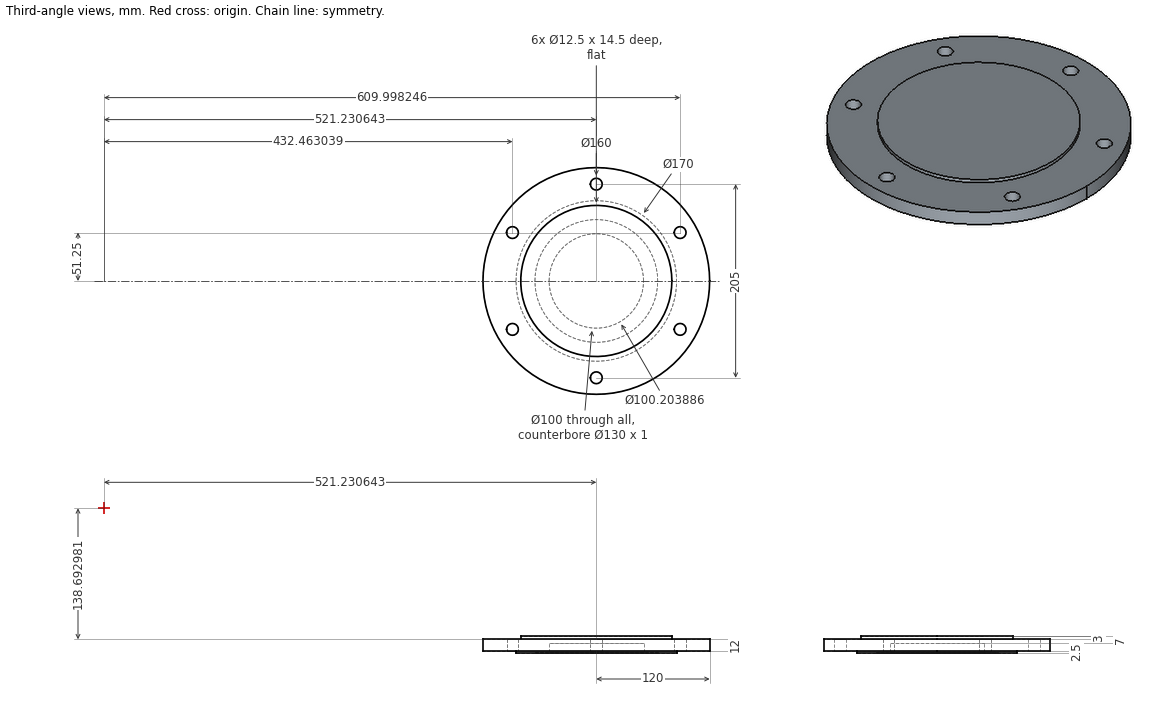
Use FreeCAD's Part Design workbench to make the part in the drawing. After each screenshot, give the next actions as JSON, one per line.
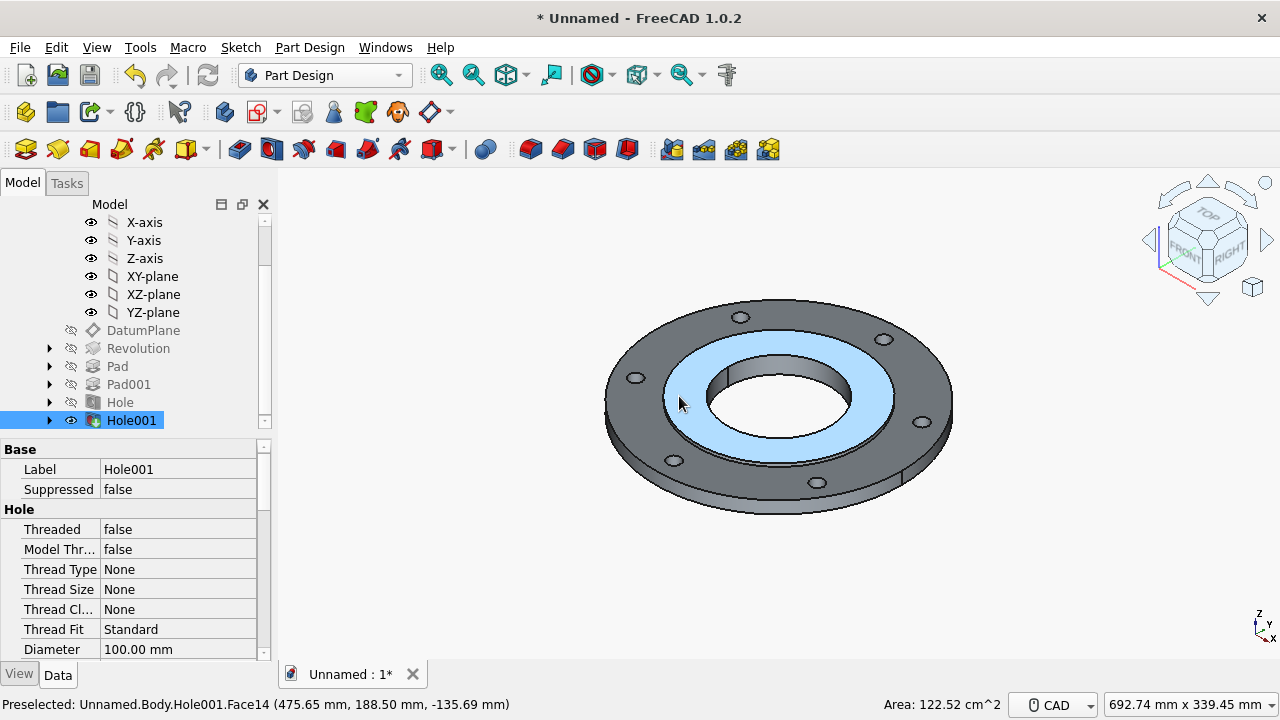
{"action": "left_click", "coordinate": [258, 112]}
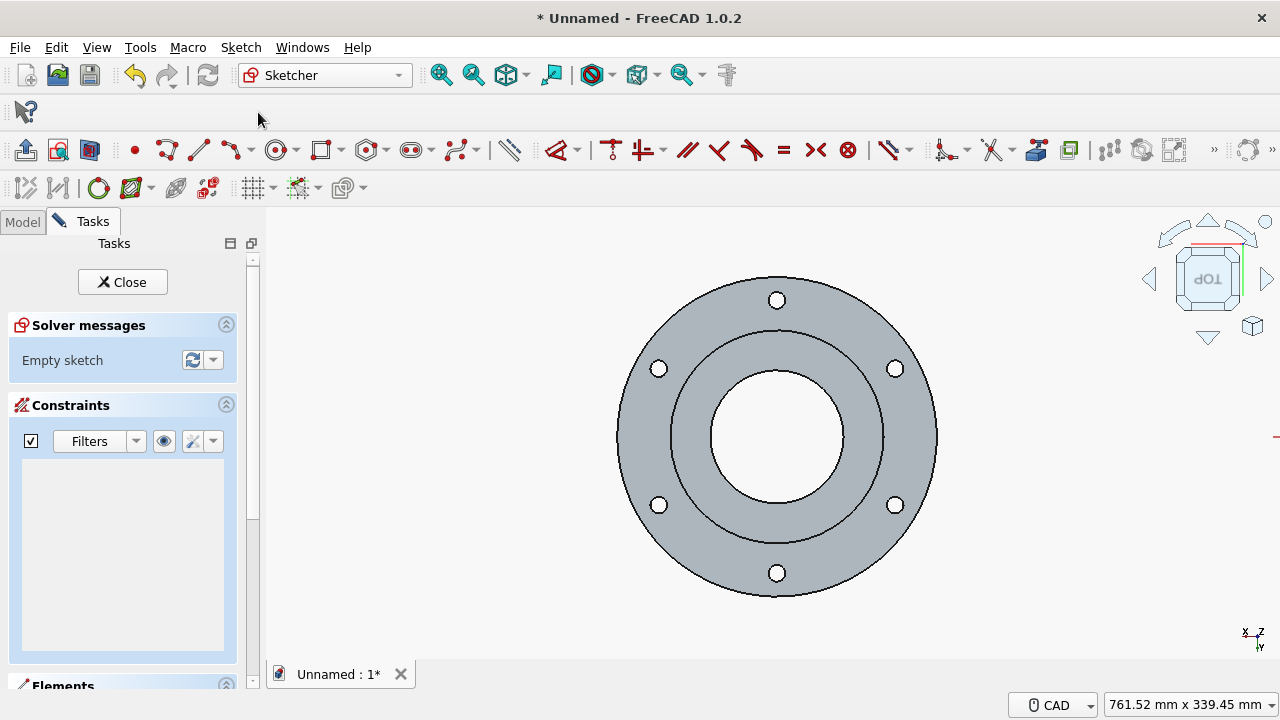
{"action": "scroll", "coordinate": [836, 440], "scroll_direction": "up", "scroll_amount": 4}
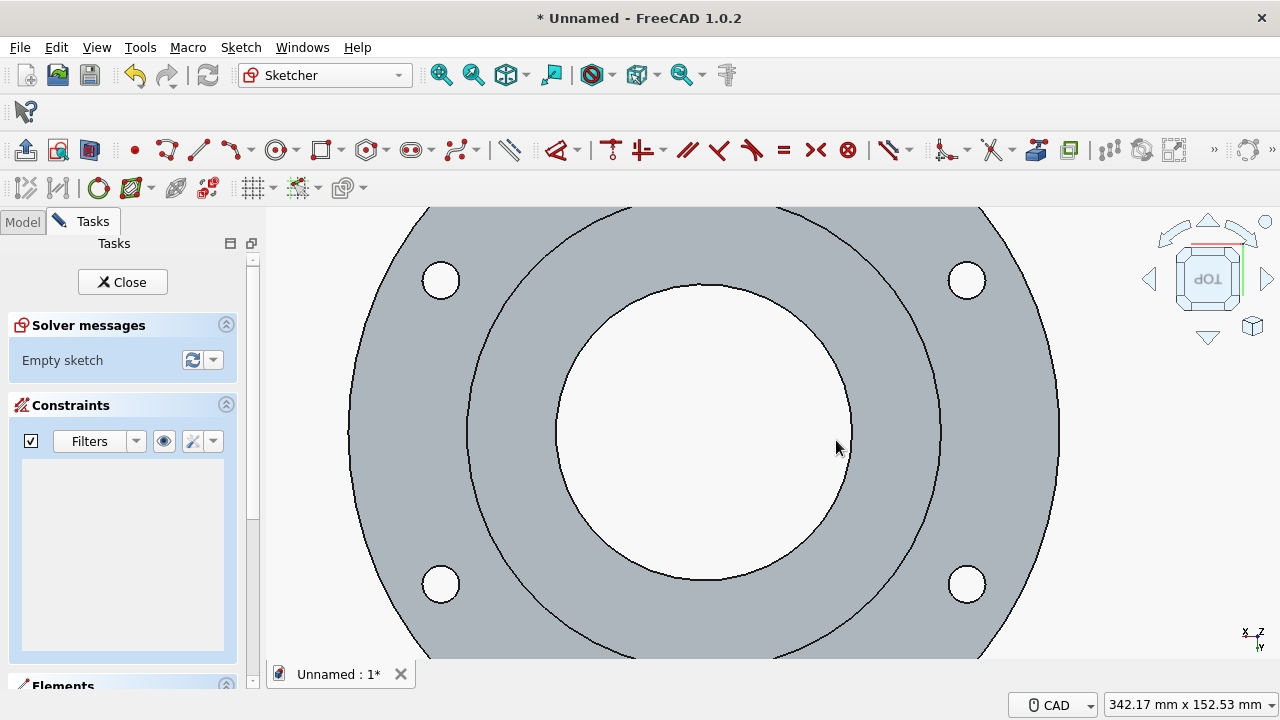
{"action": "key", "text": "g c"}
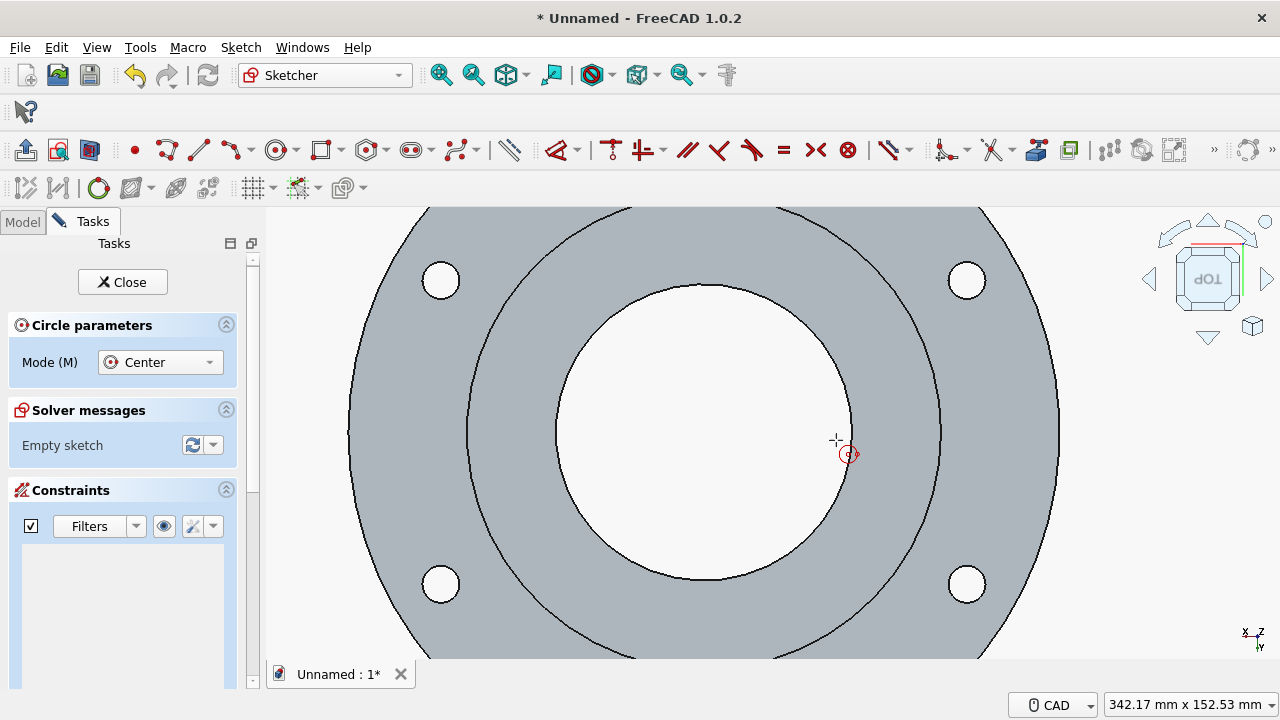
{"action": "left_click", "coordinate": [704, 432]}
{"action": "mouse_move", "coordinate": [809, 327]}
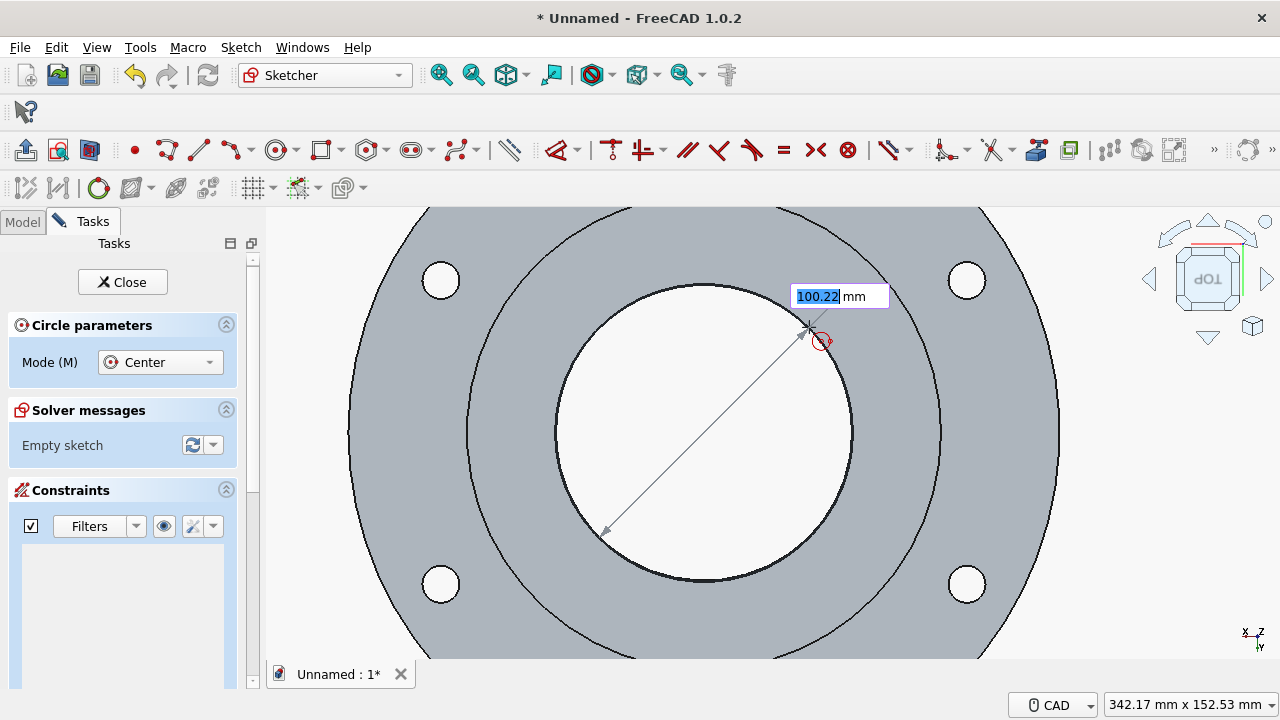
{"action": "type", "text": "100.203886"}
{"action": "key", "text": "Return"}
{"action": "key", "text": "Escape"}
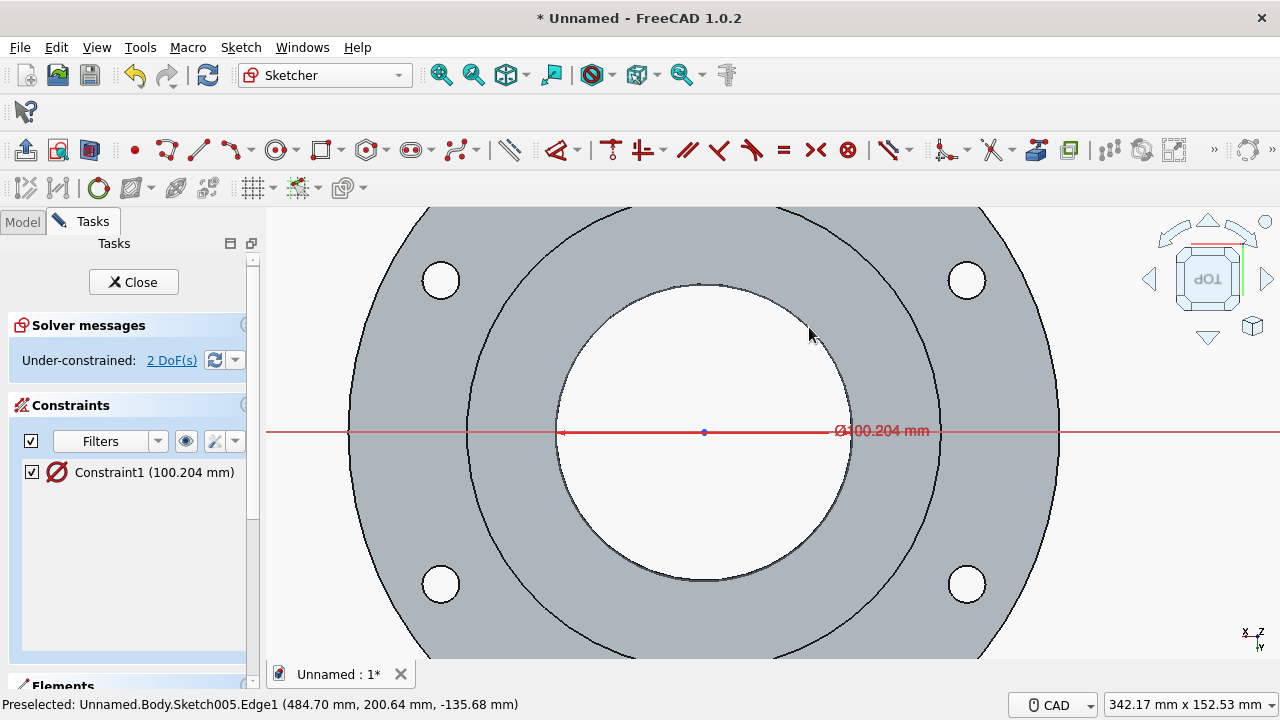
{"action": "left_click", "coordinate": [704, 433]}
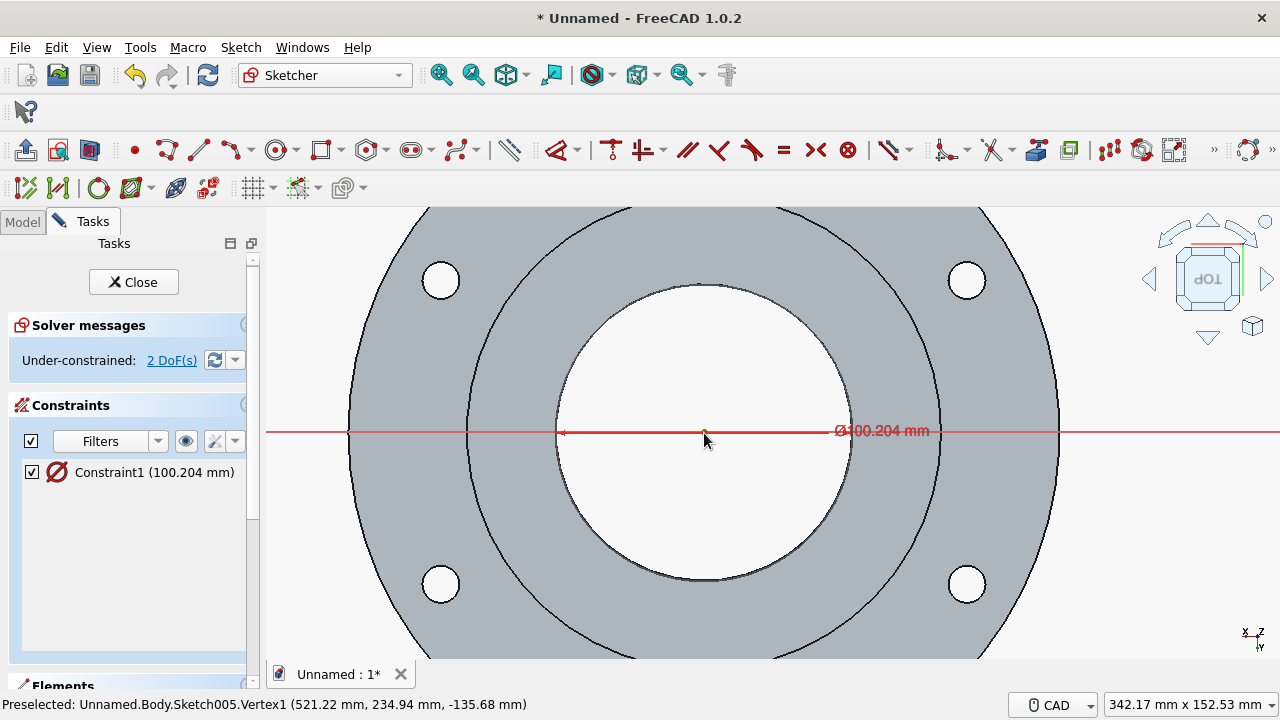
{"action": "left_click", "coordinate": [353, 432]}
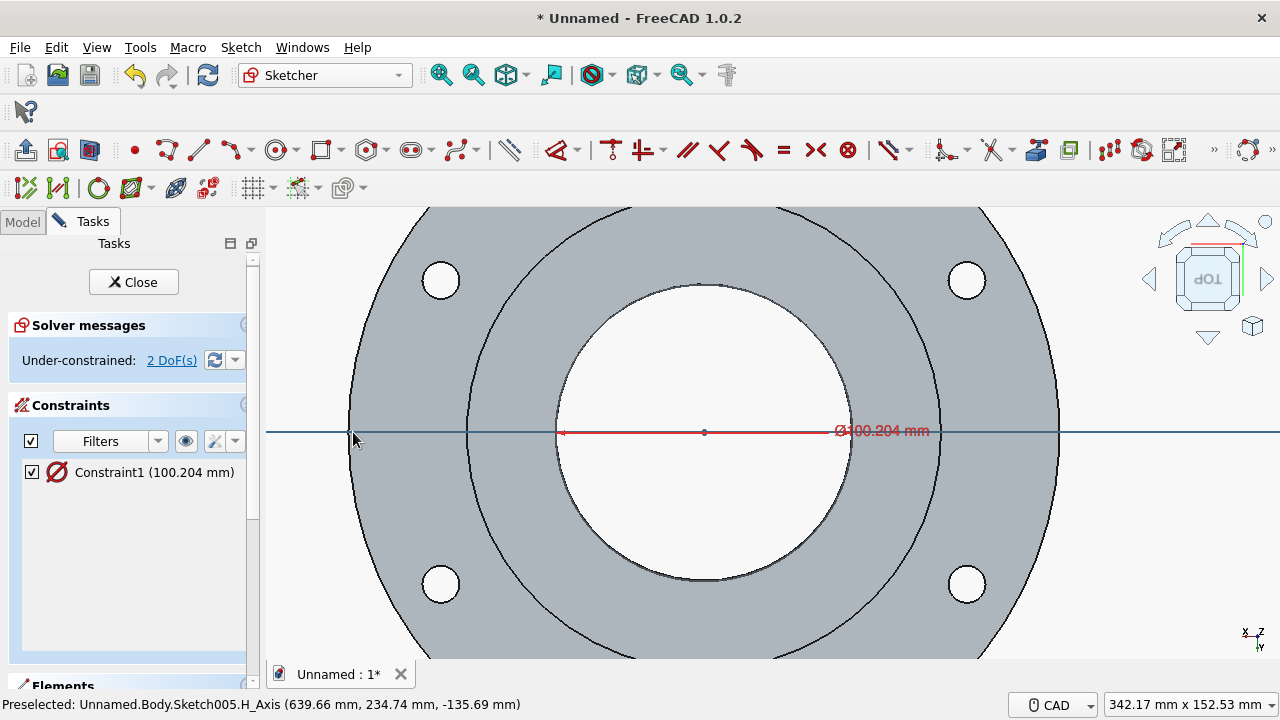
{"action": "key", "text": "c"}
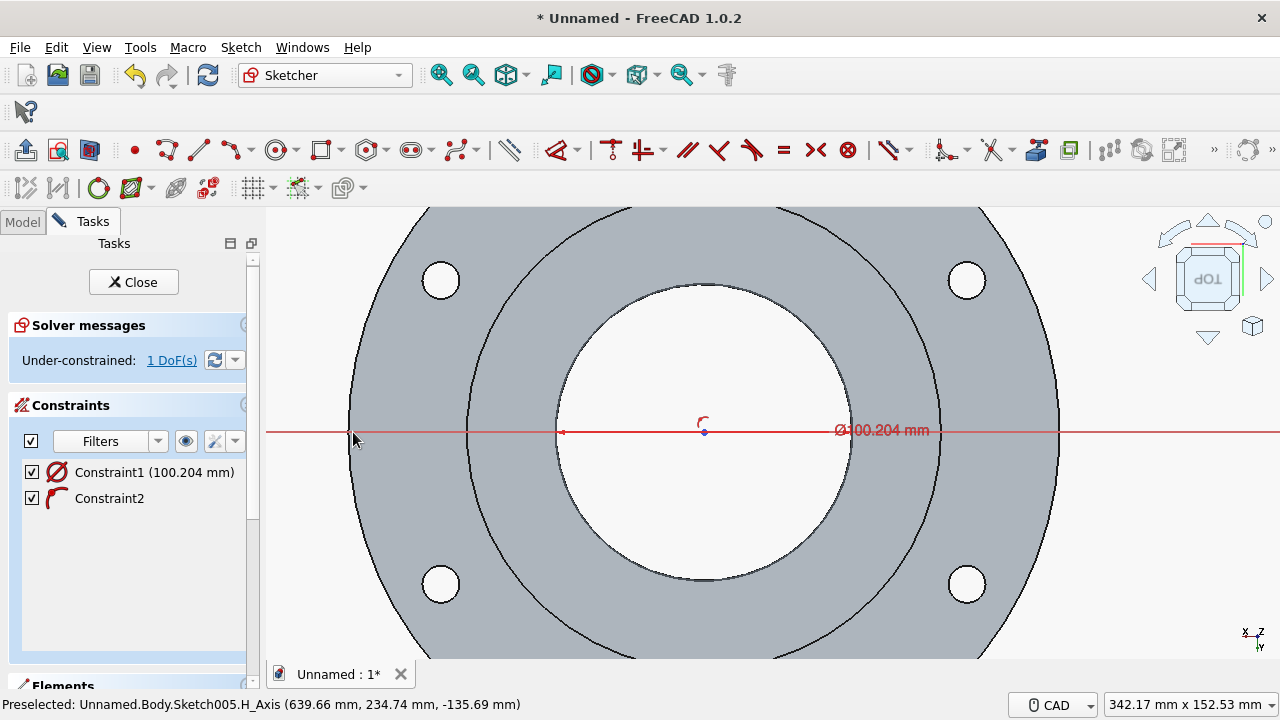
{"action": "key", "text": "d"}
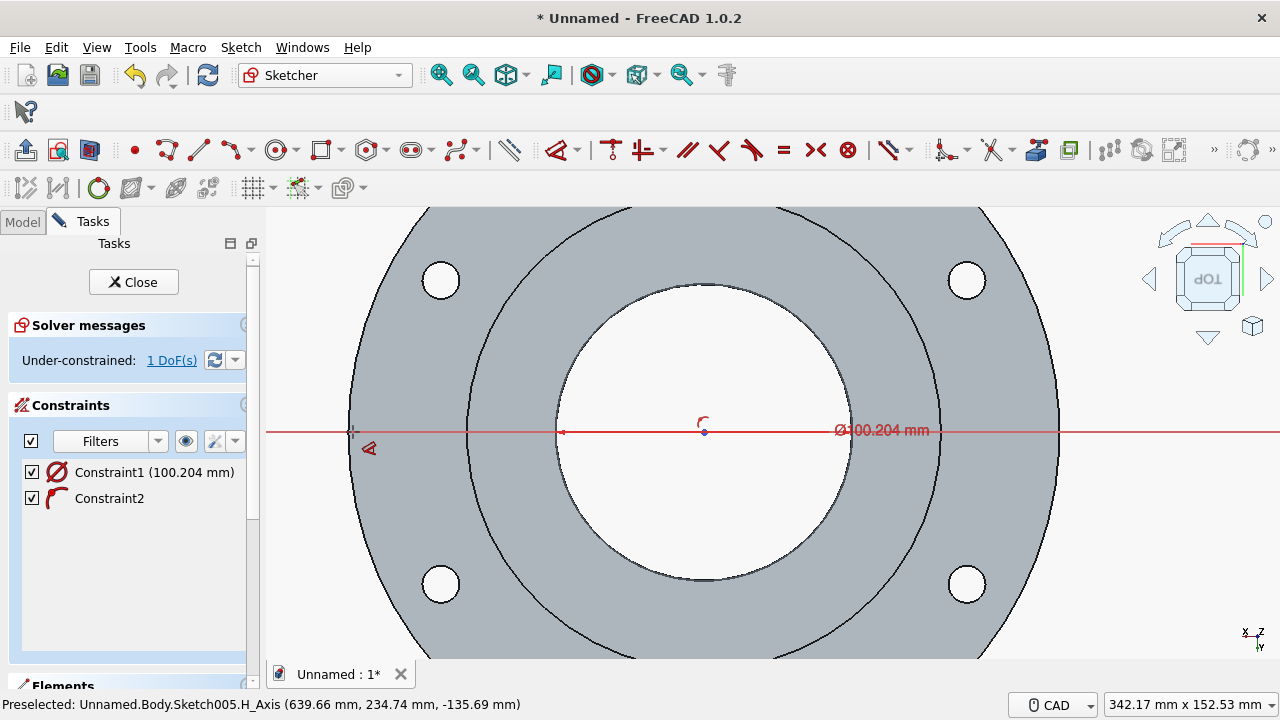
{"action": "left_click", "coordinate": [704, 432]}
{"action": "left_click", "coordinate": [909, 466]}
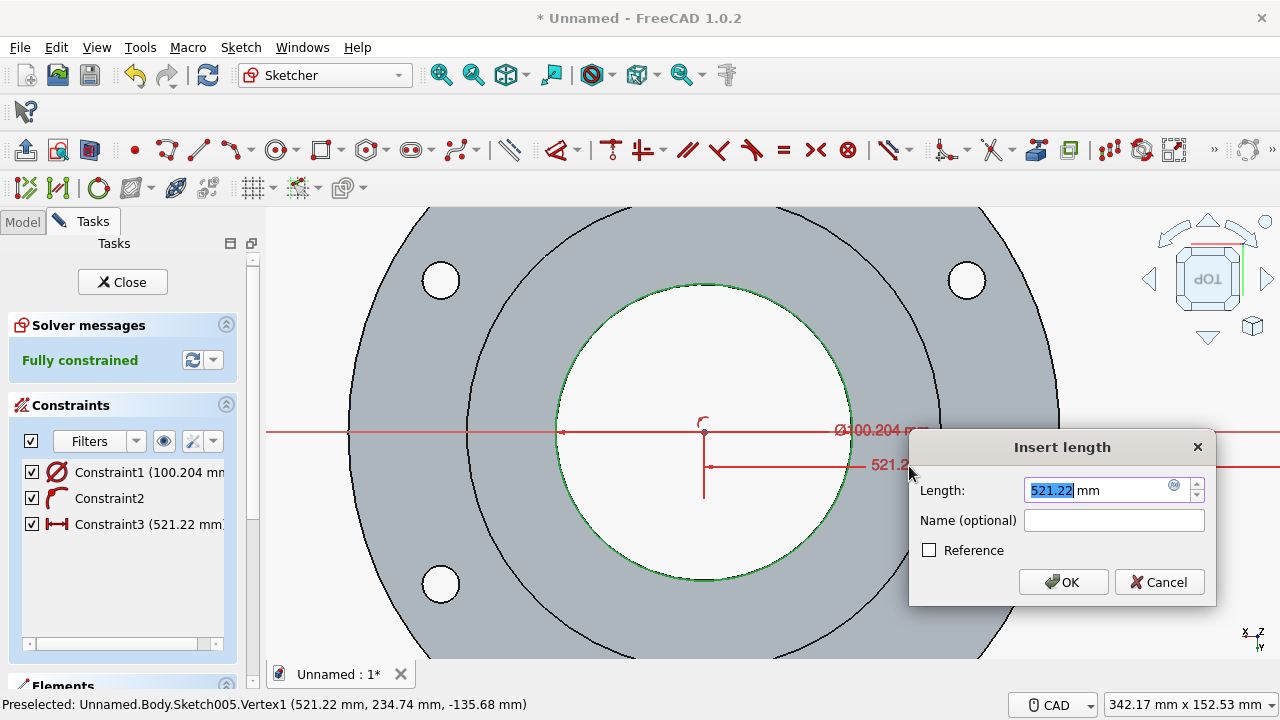
{"action": "type", "text": "521.230643"}
{"action": "key", "text": "Return"}
{"action": "key", "text": "Escape"}